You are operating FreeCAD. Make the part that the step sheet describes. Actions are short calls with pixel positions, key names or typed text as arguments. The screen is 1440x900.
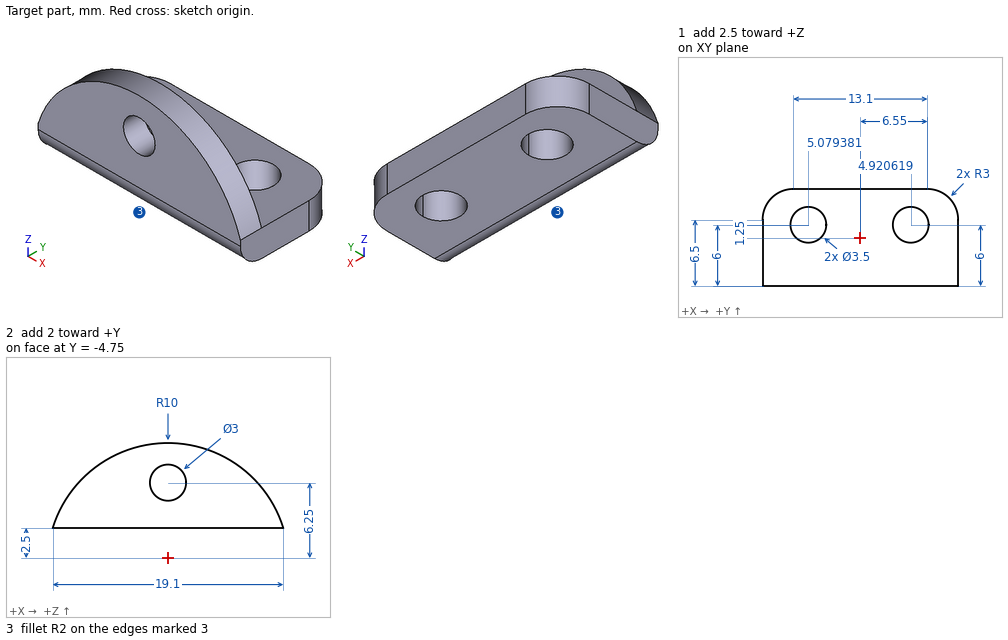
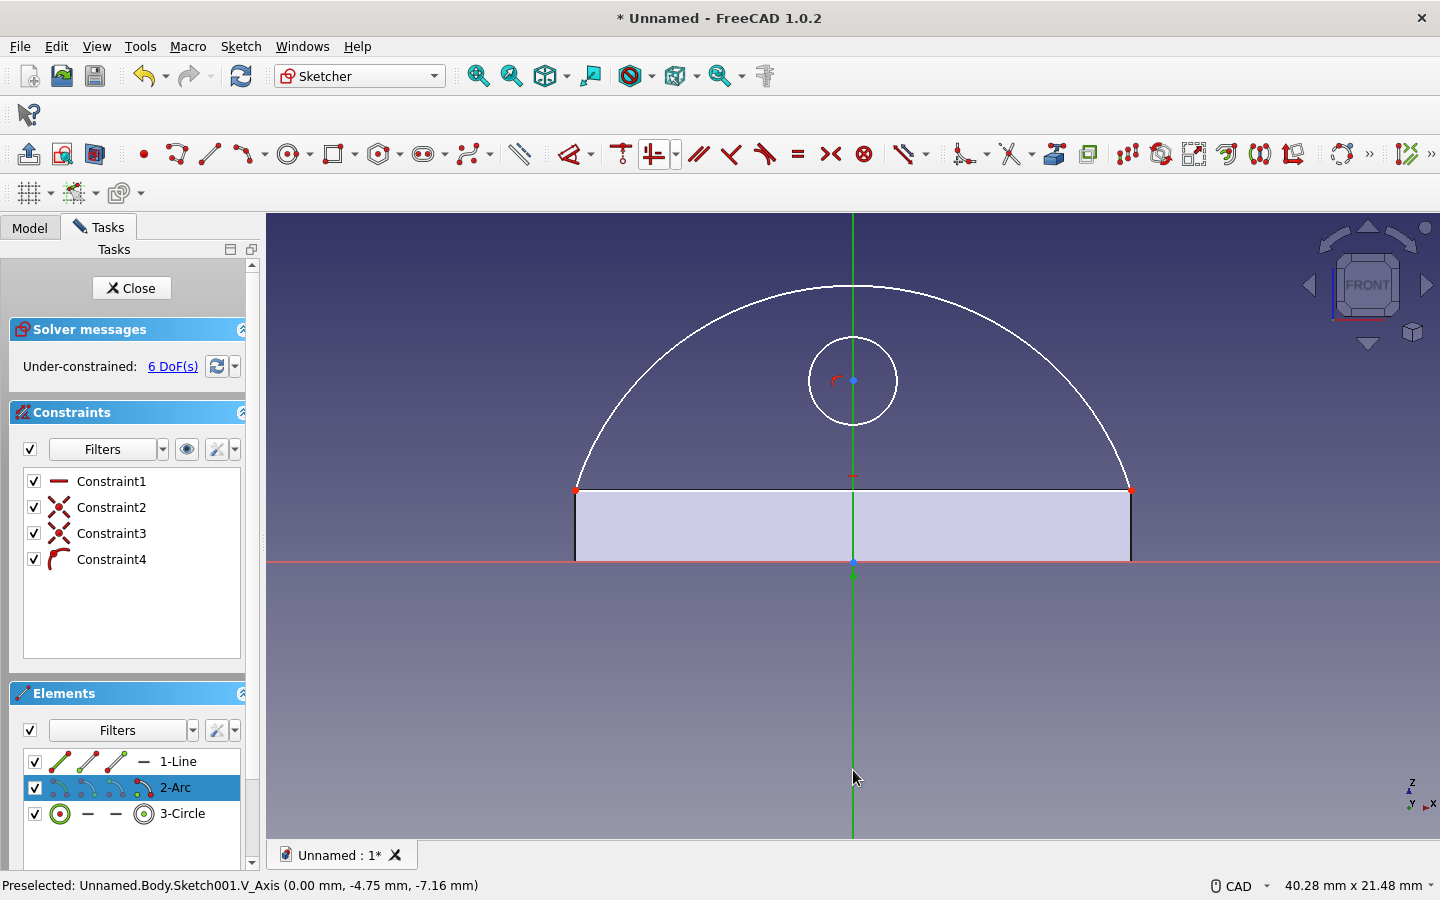
click(621, 154)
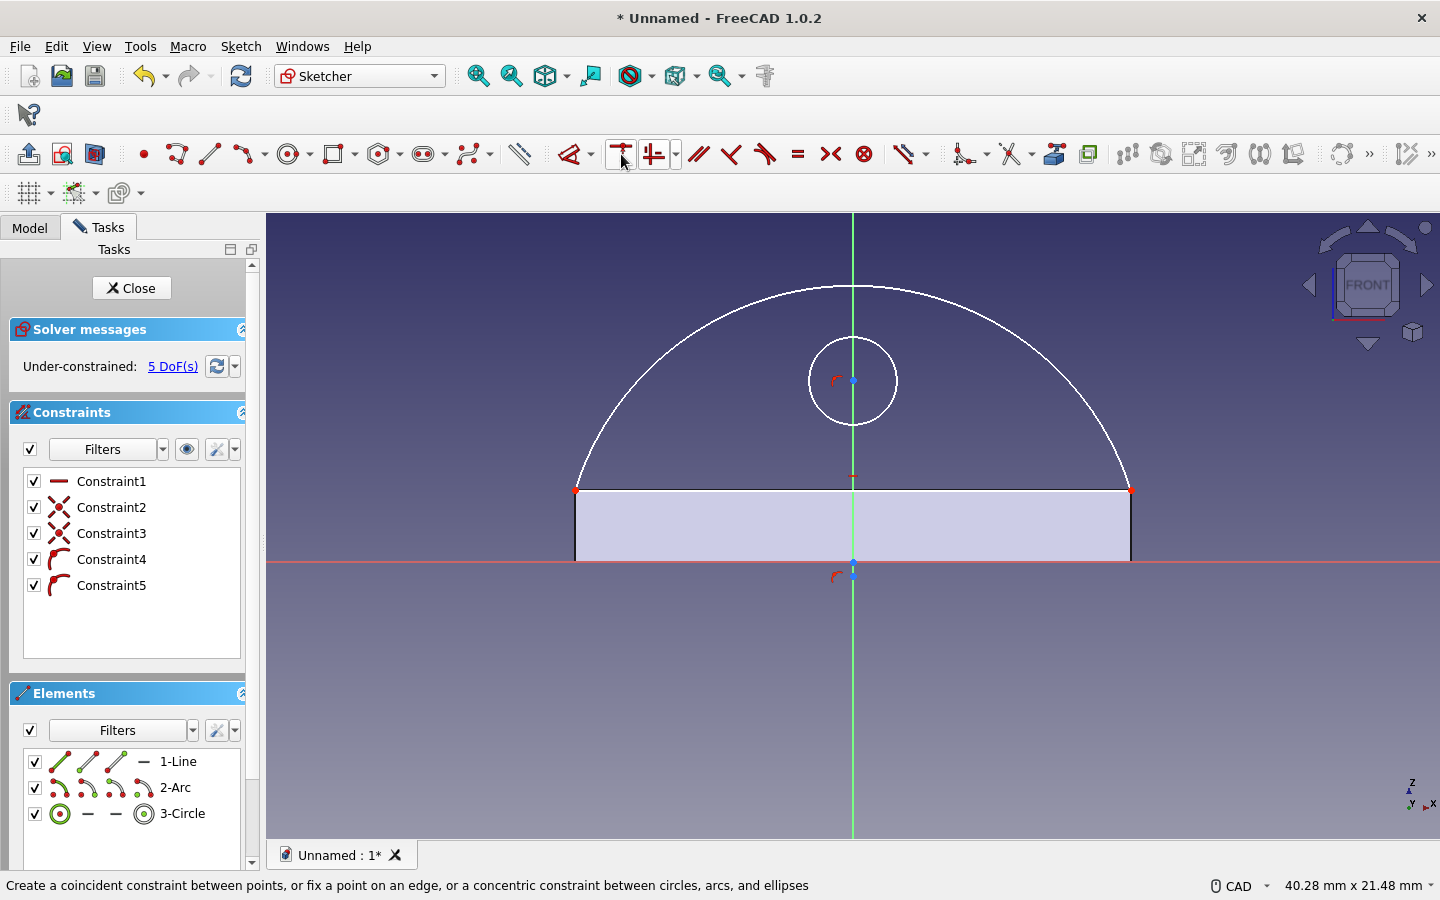
click(568, 154)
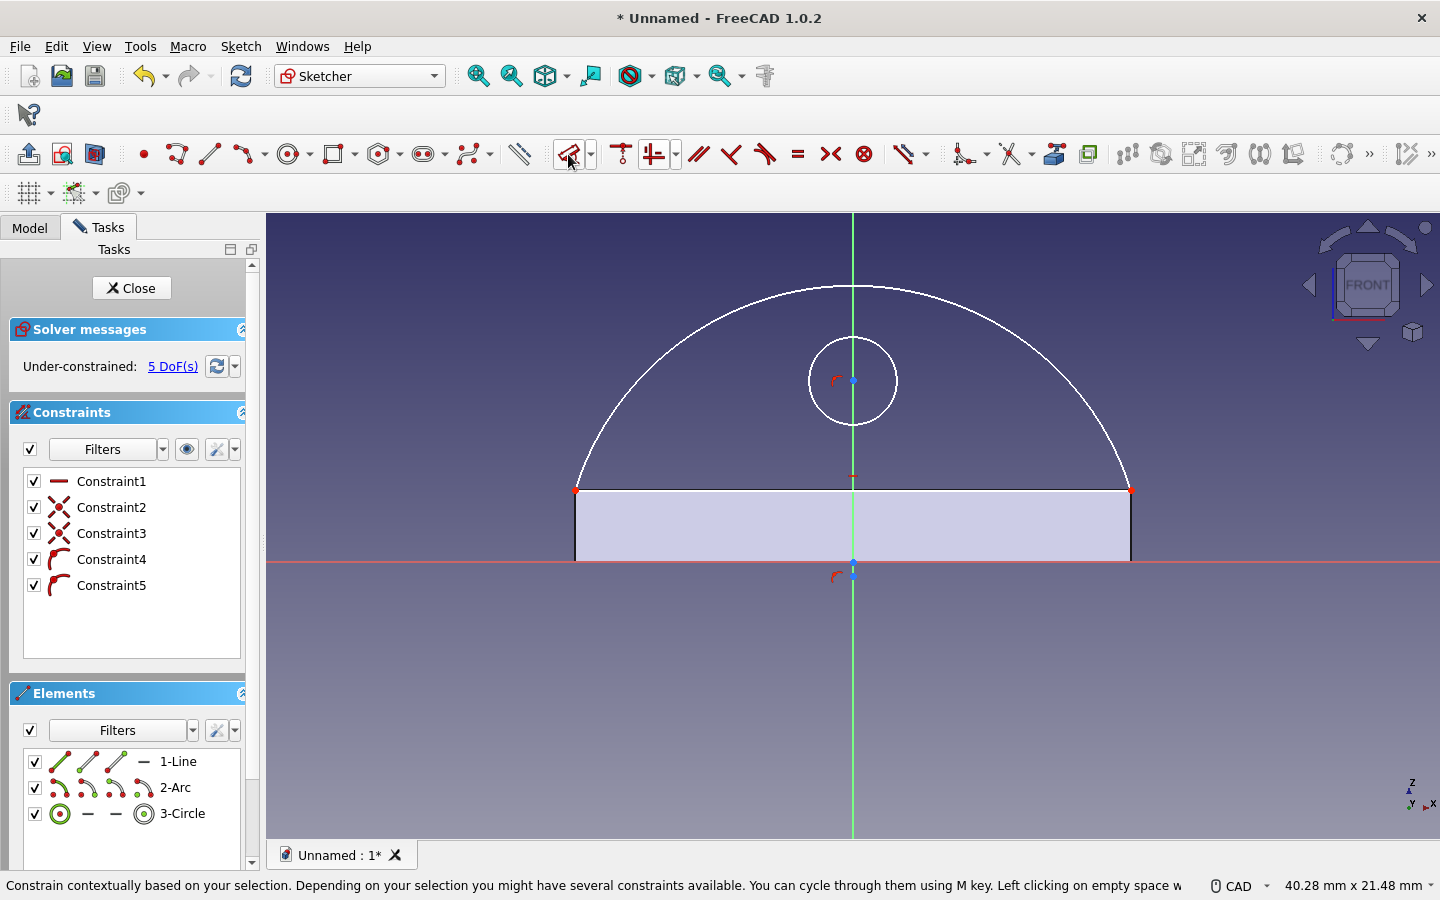
click(995, 323)
click(1011, 295)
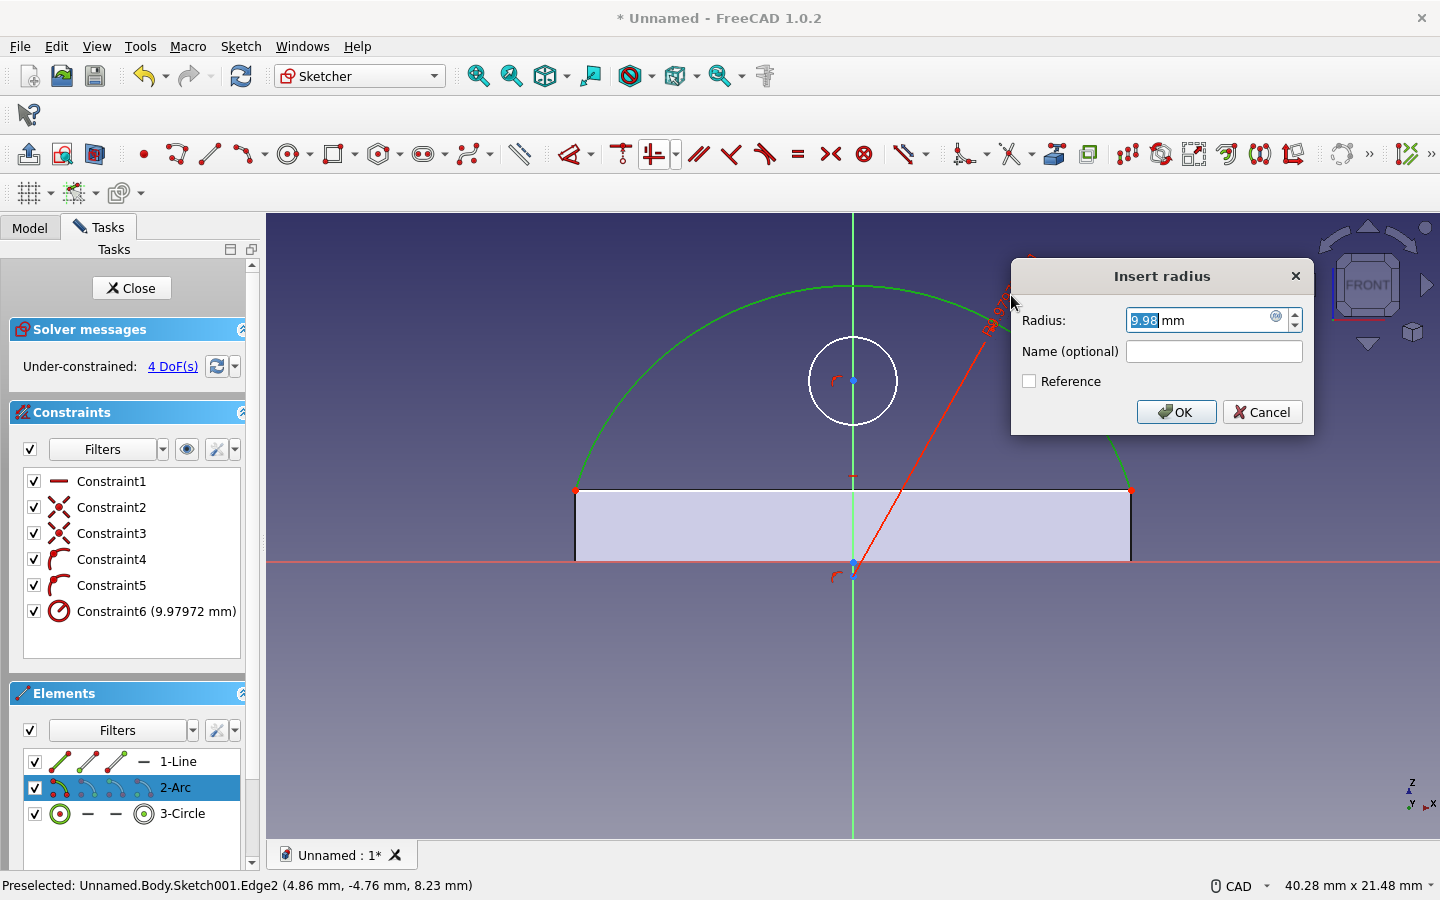
text(10)
key(Return)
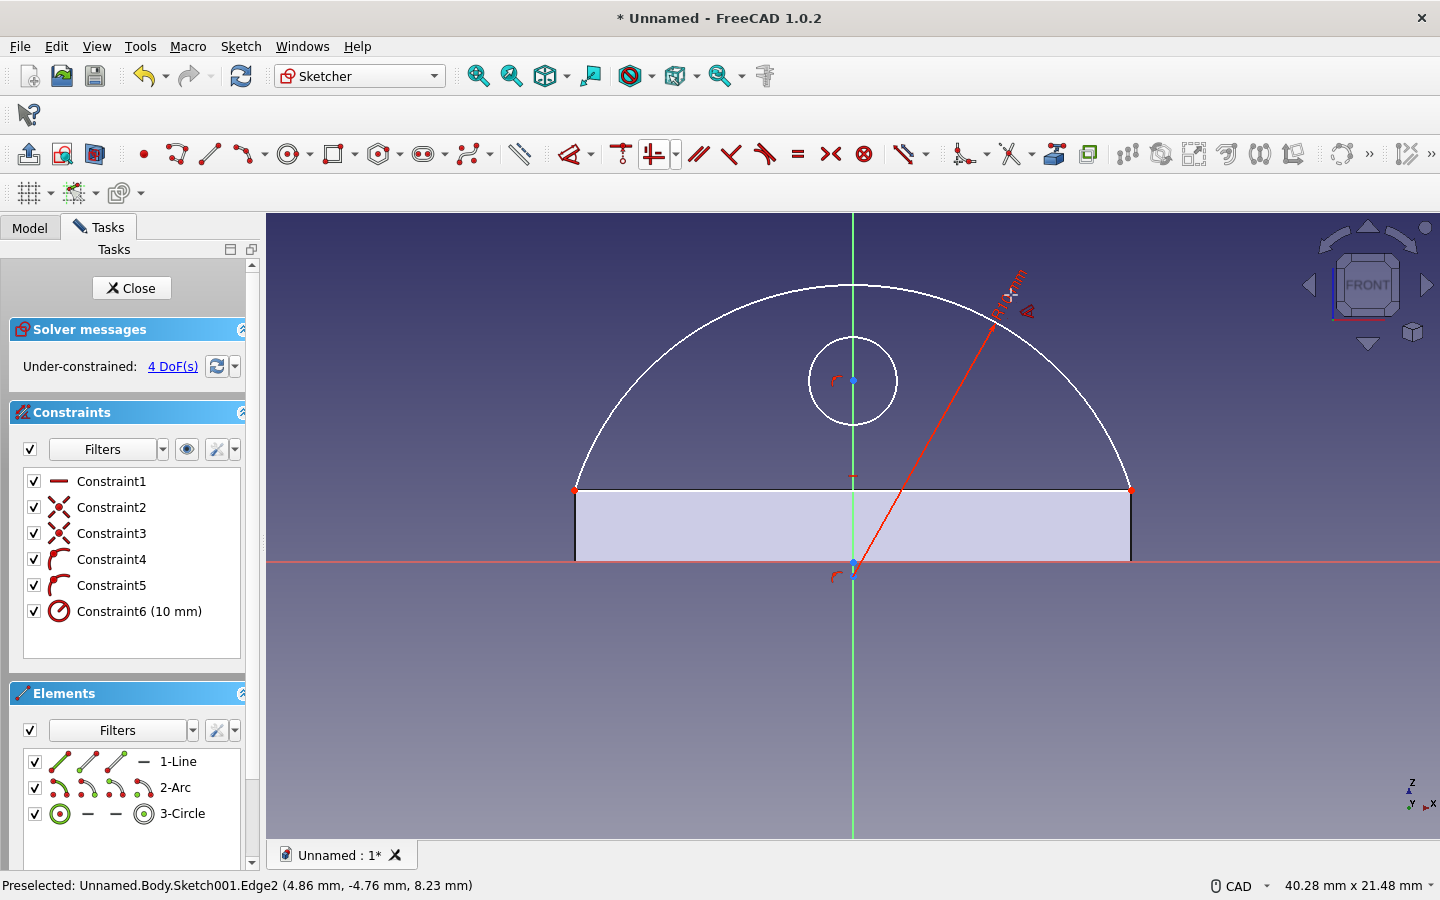
click(884, 350)
click(907, 327)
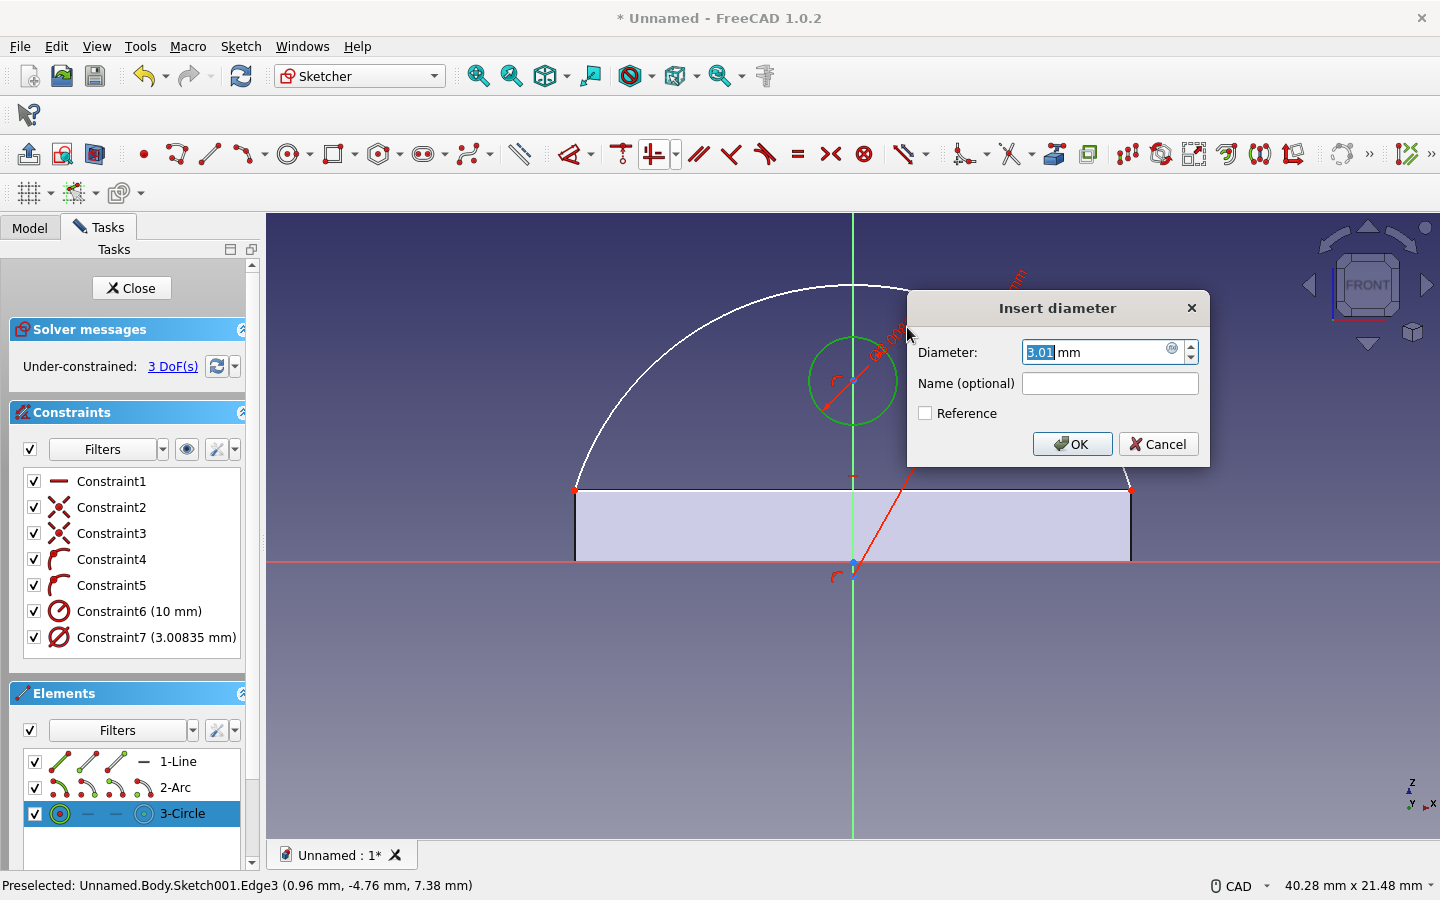
text(3)
key(Return)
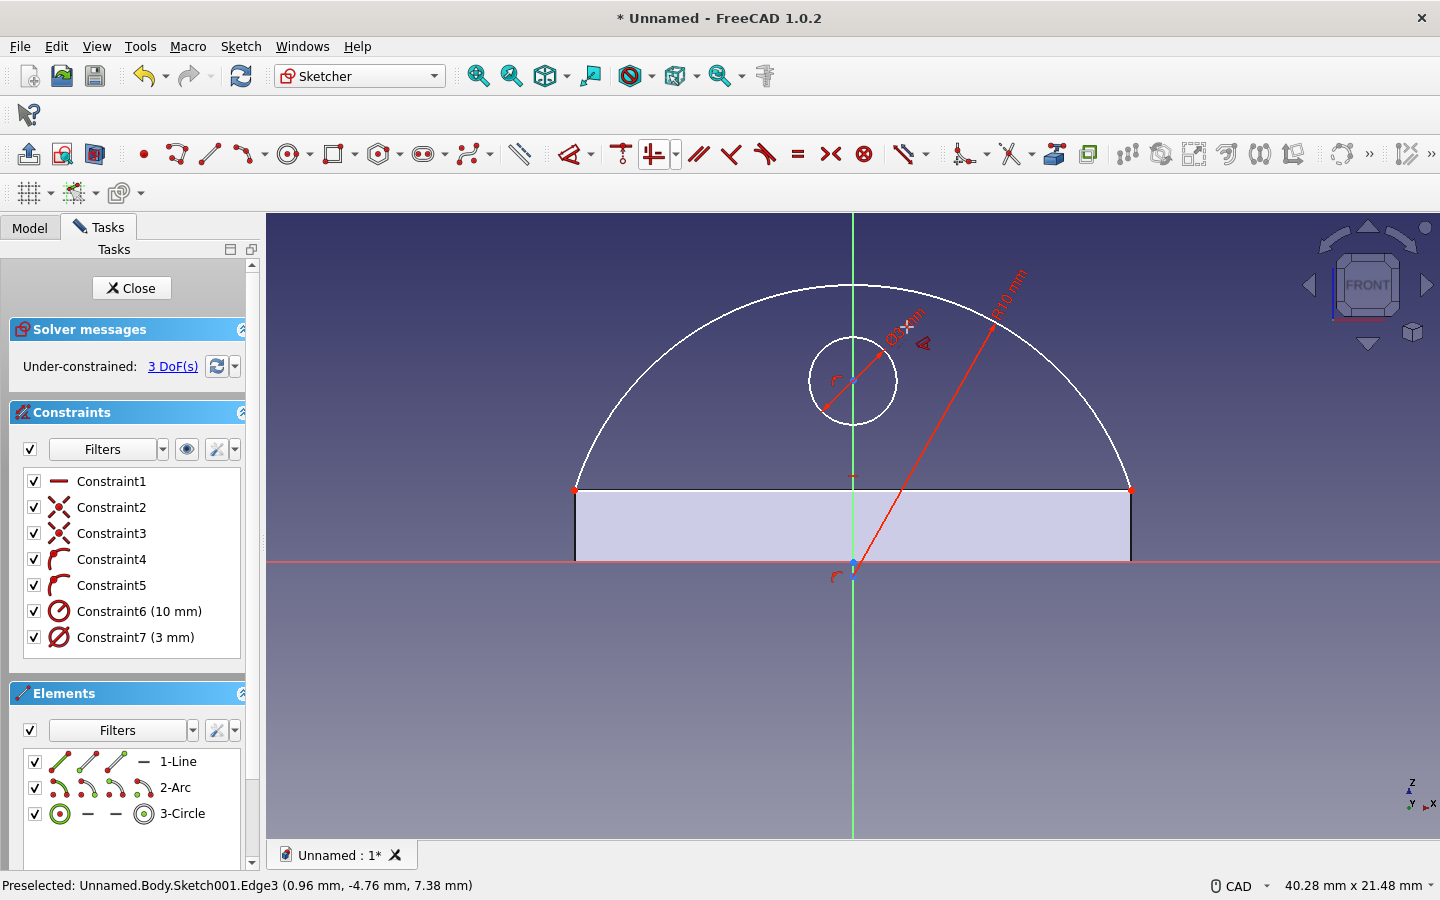
click(742, 491)
click(725, 525)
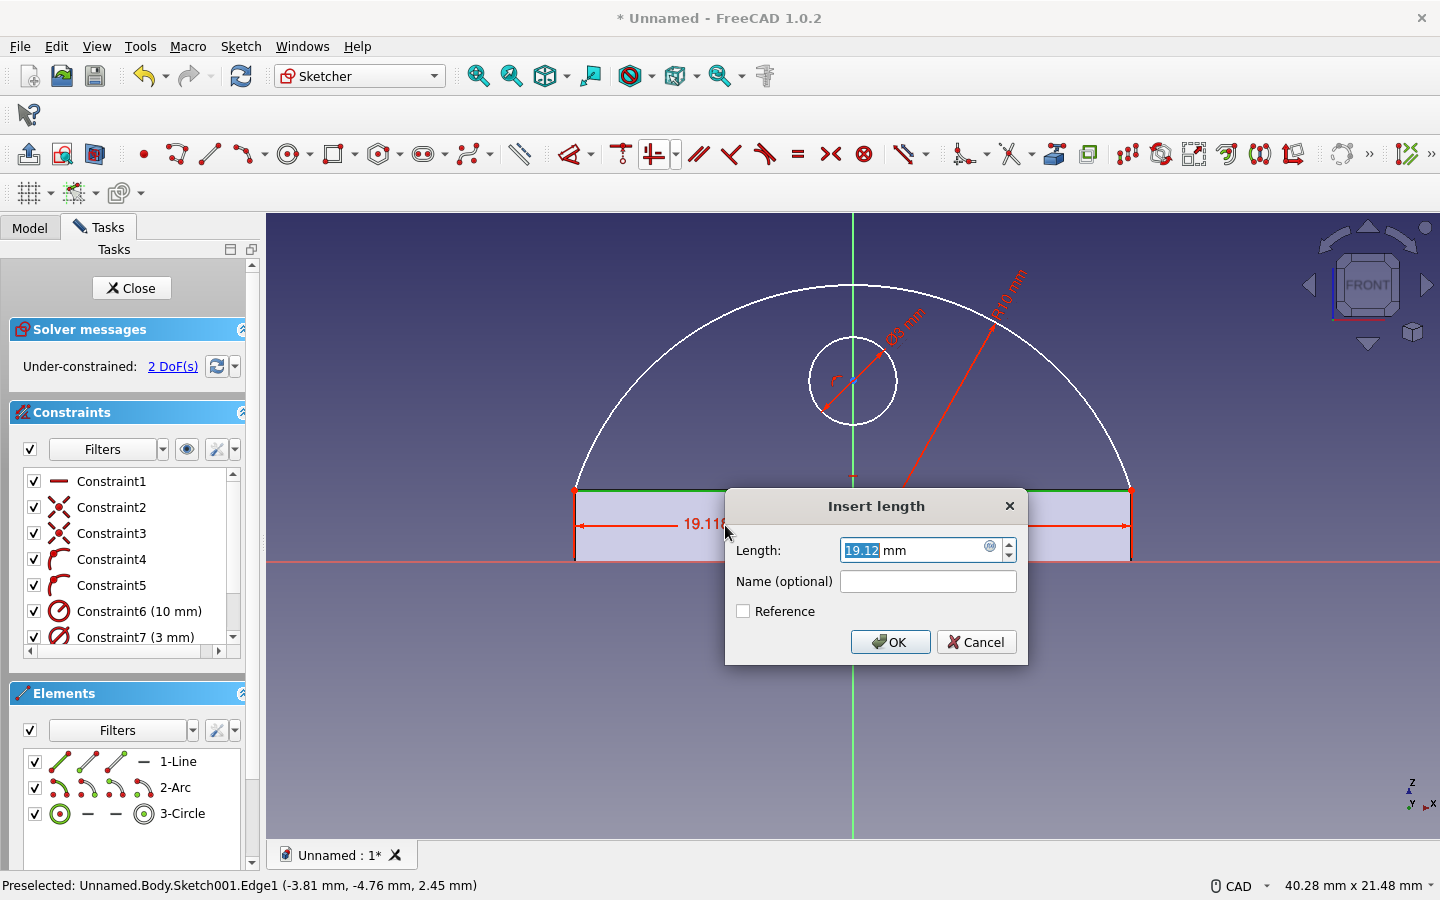
text(19.1)
key(Return)